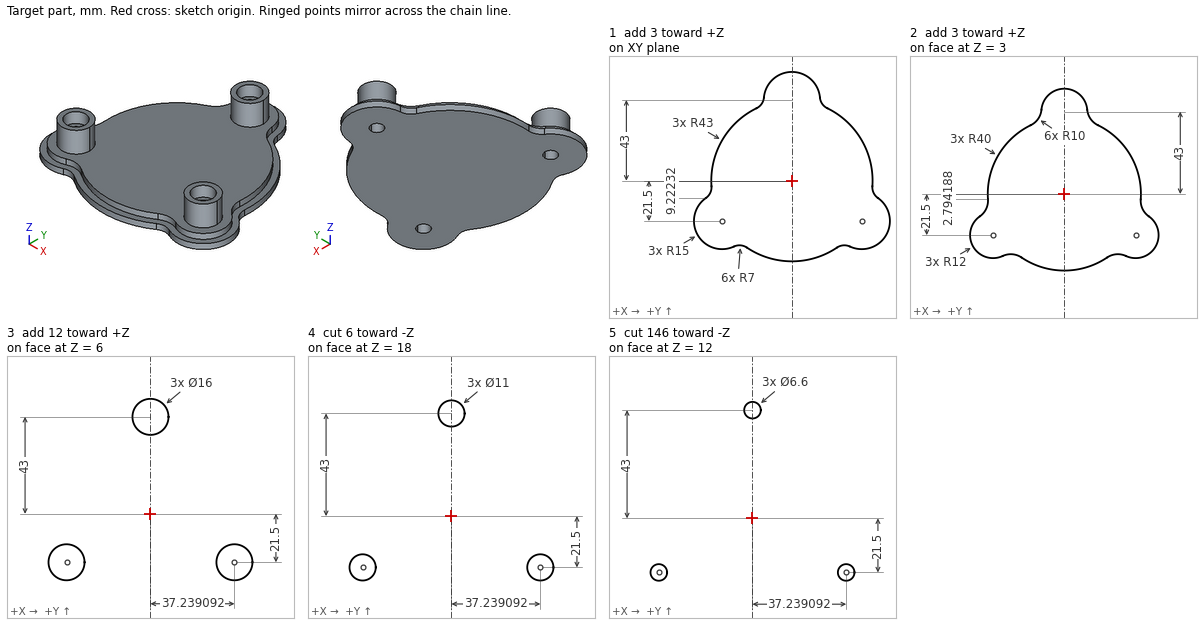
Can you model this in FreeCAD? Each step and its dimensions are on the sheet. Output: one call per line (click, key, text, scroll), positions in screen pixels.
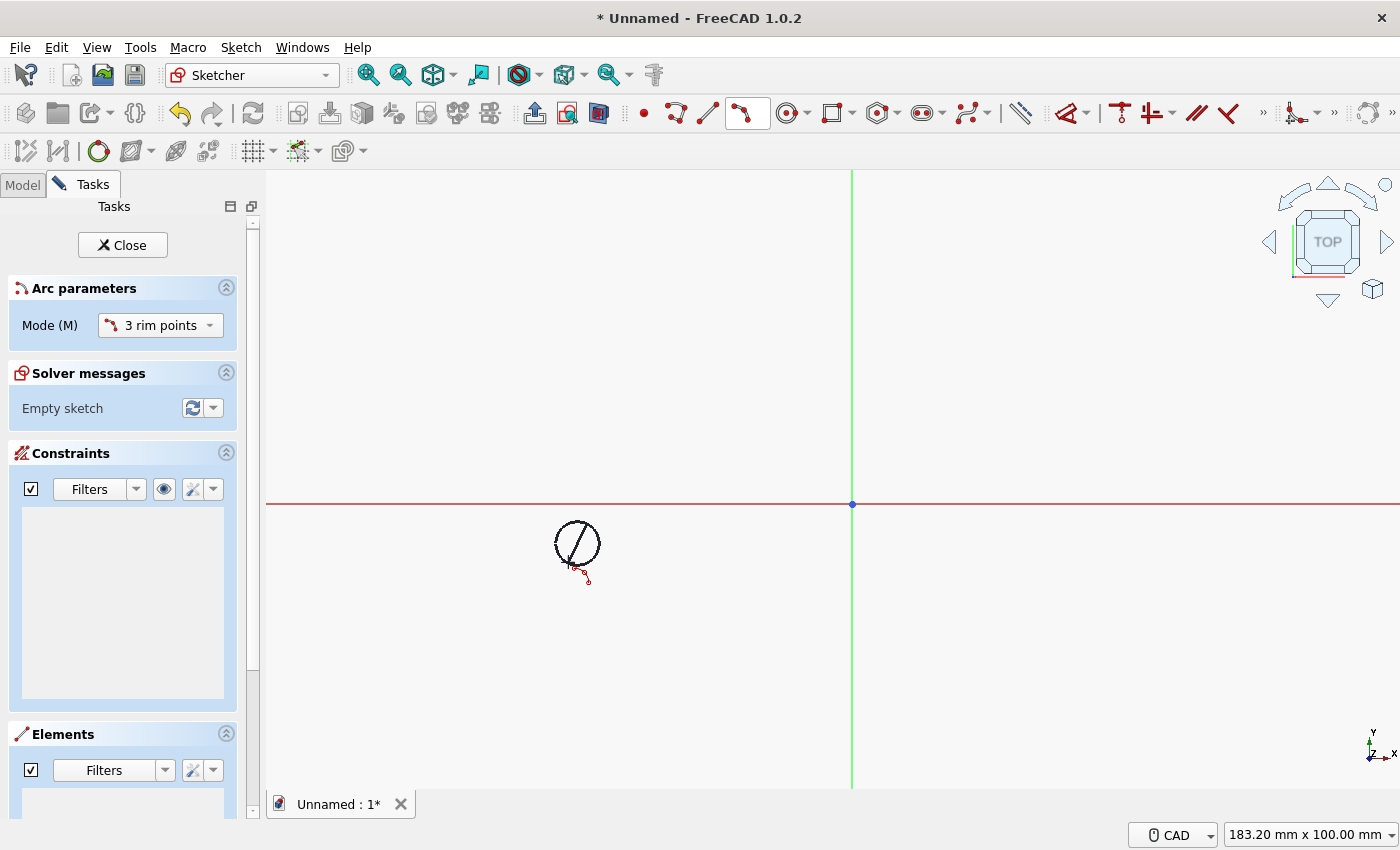
scroll(582, 545, up, 6)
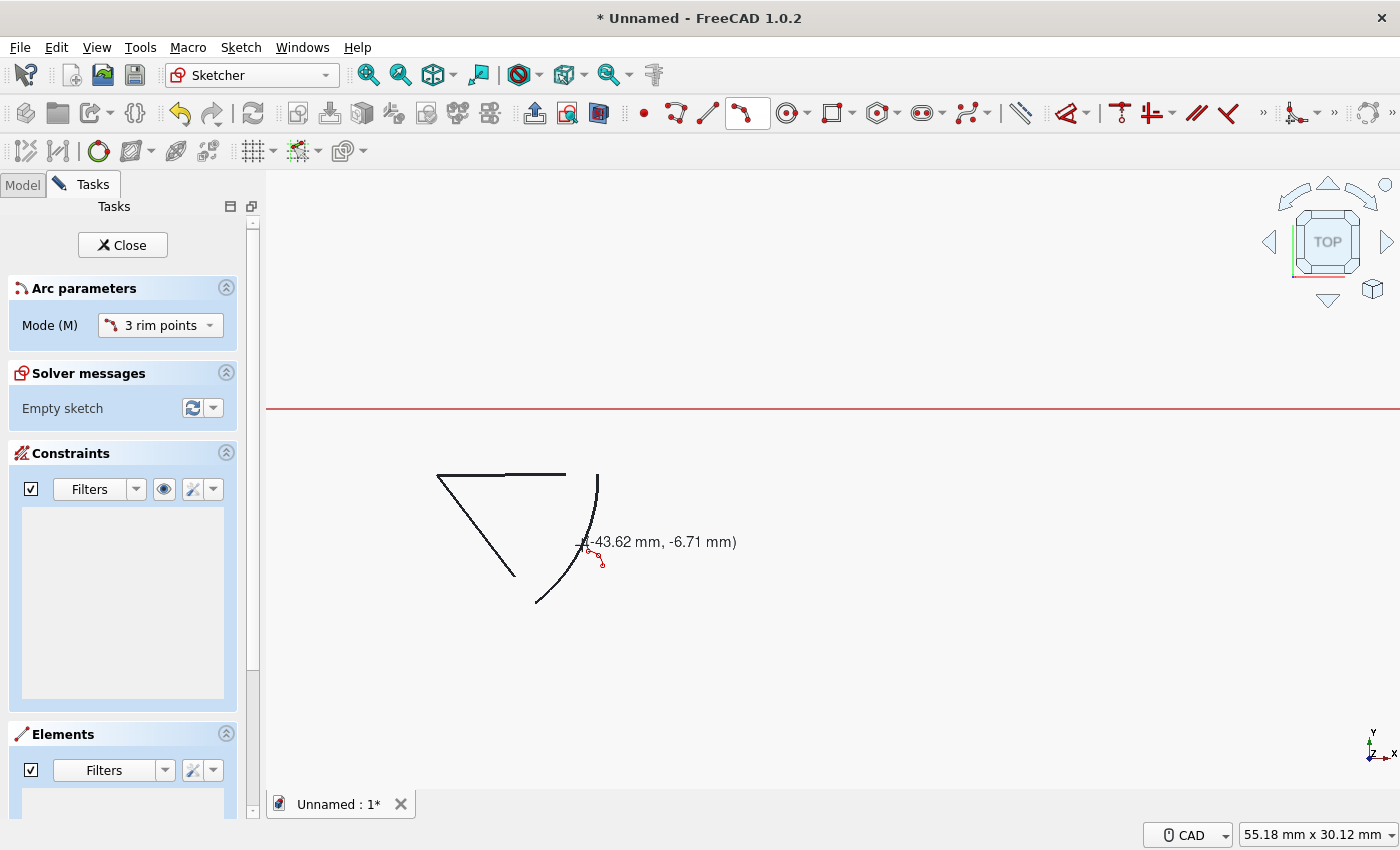
click(583, 543)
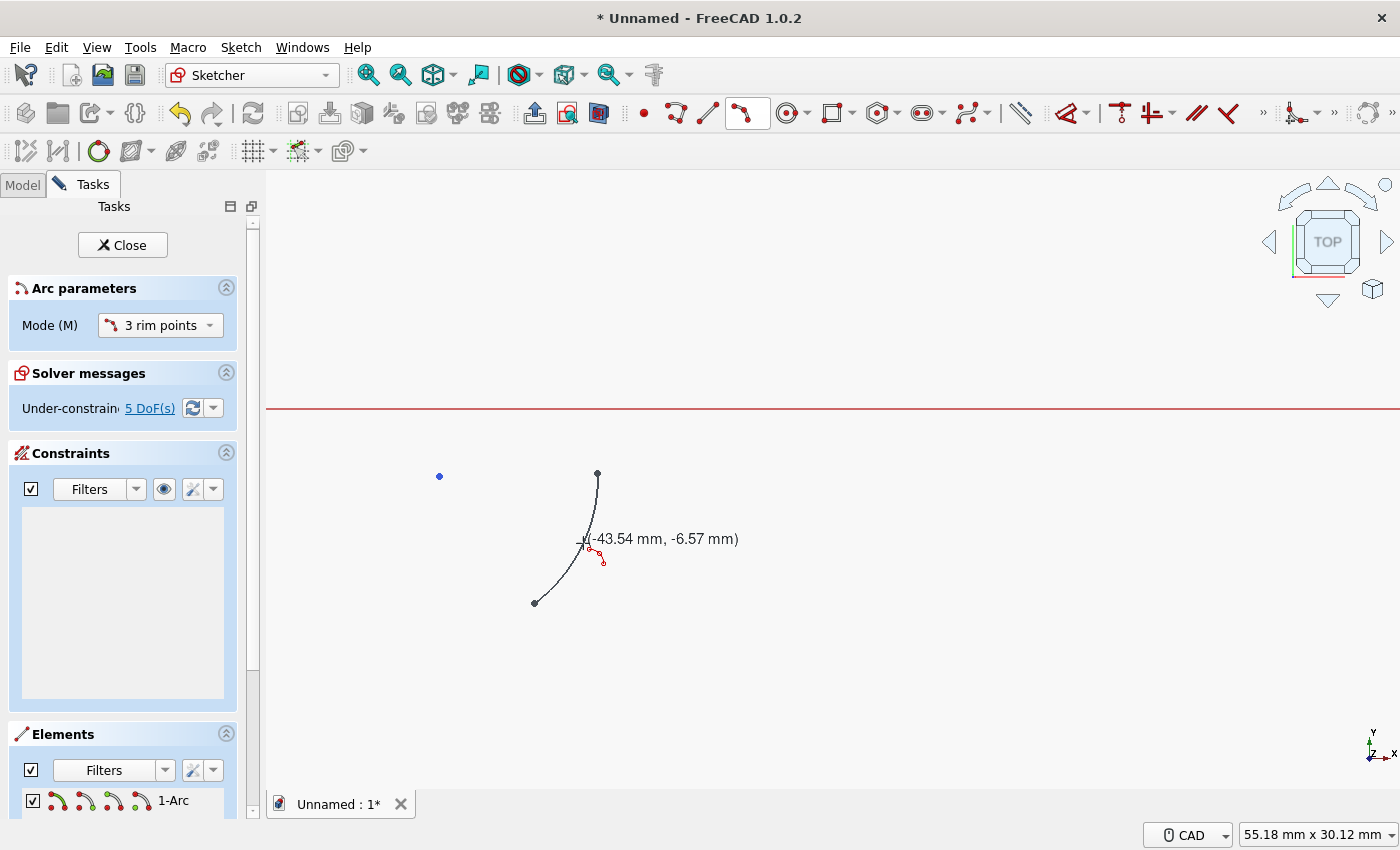
scroll(584, 536, down, 8)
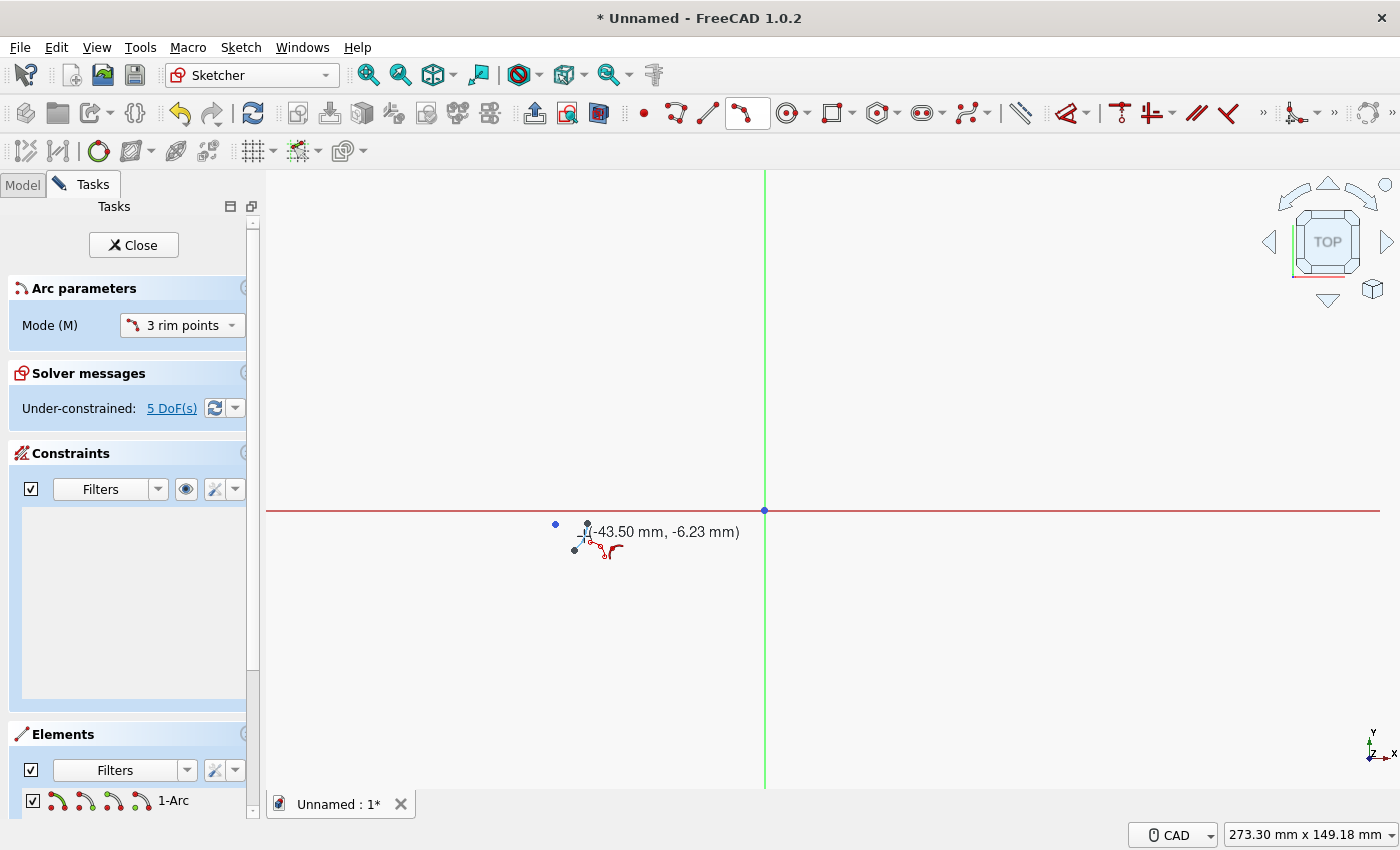
click(574, 550)
click(636, 656)
click(556, 631)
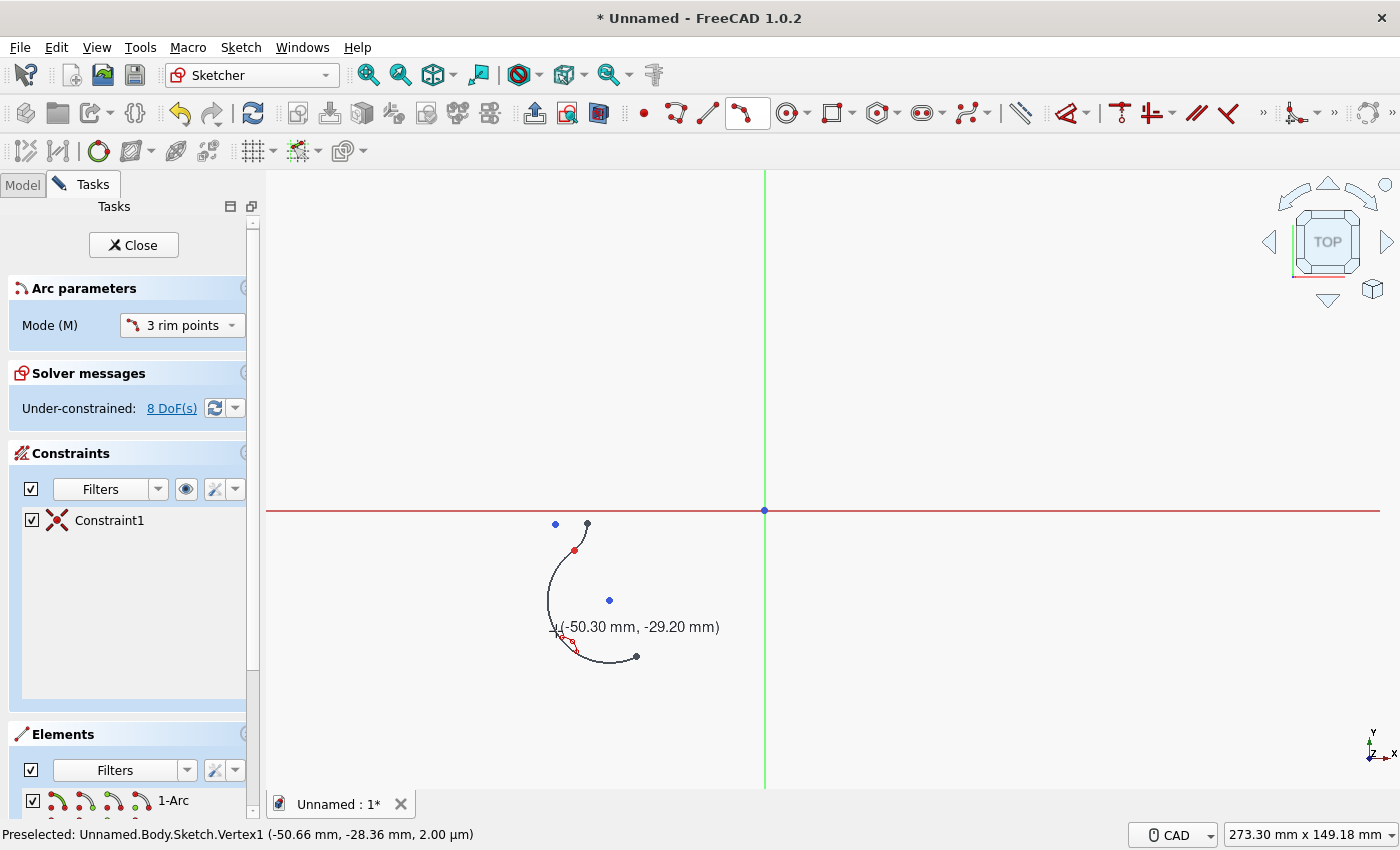
click(636, 657)
click(665, 659)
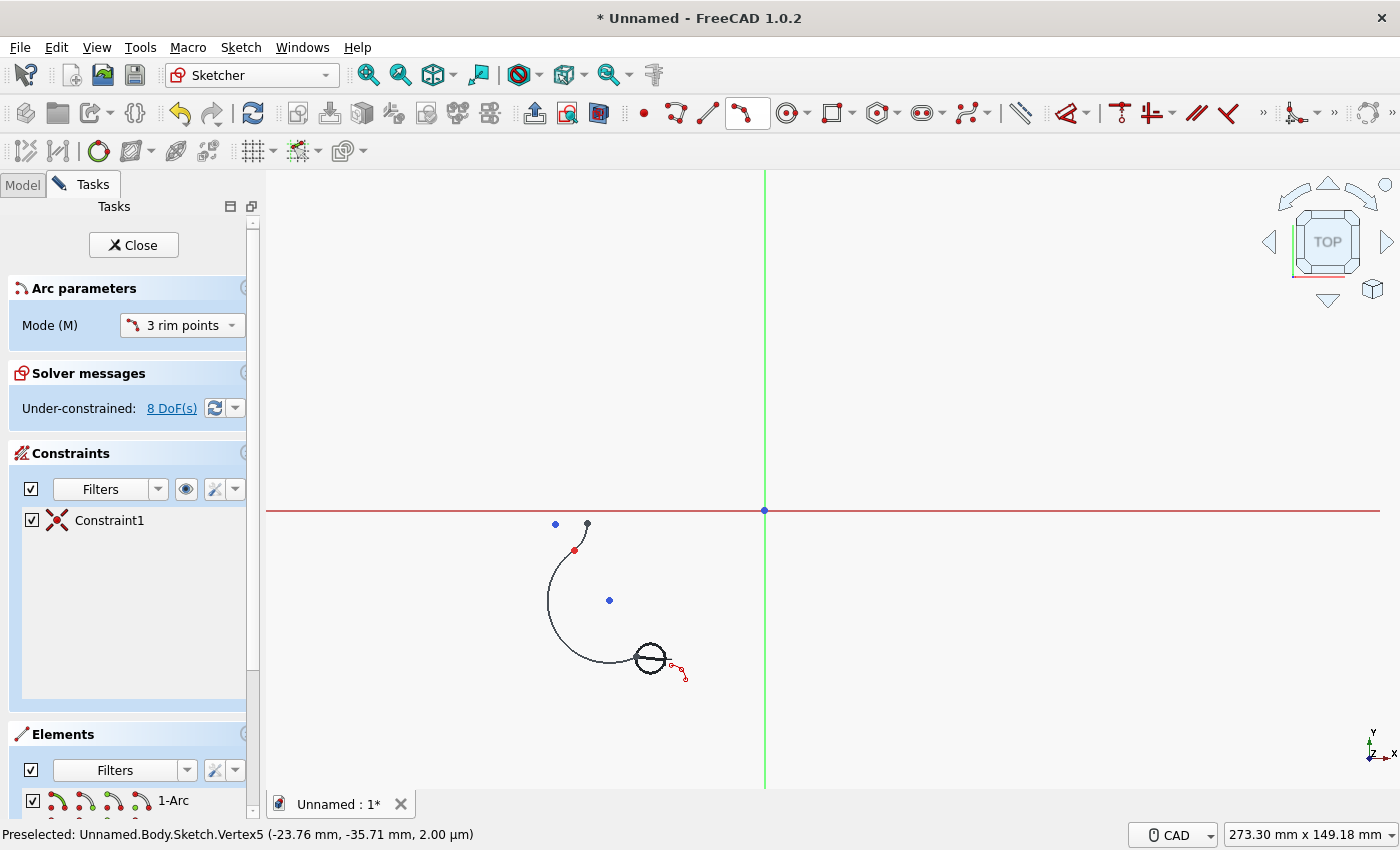
scroll(651, 654, up, 8)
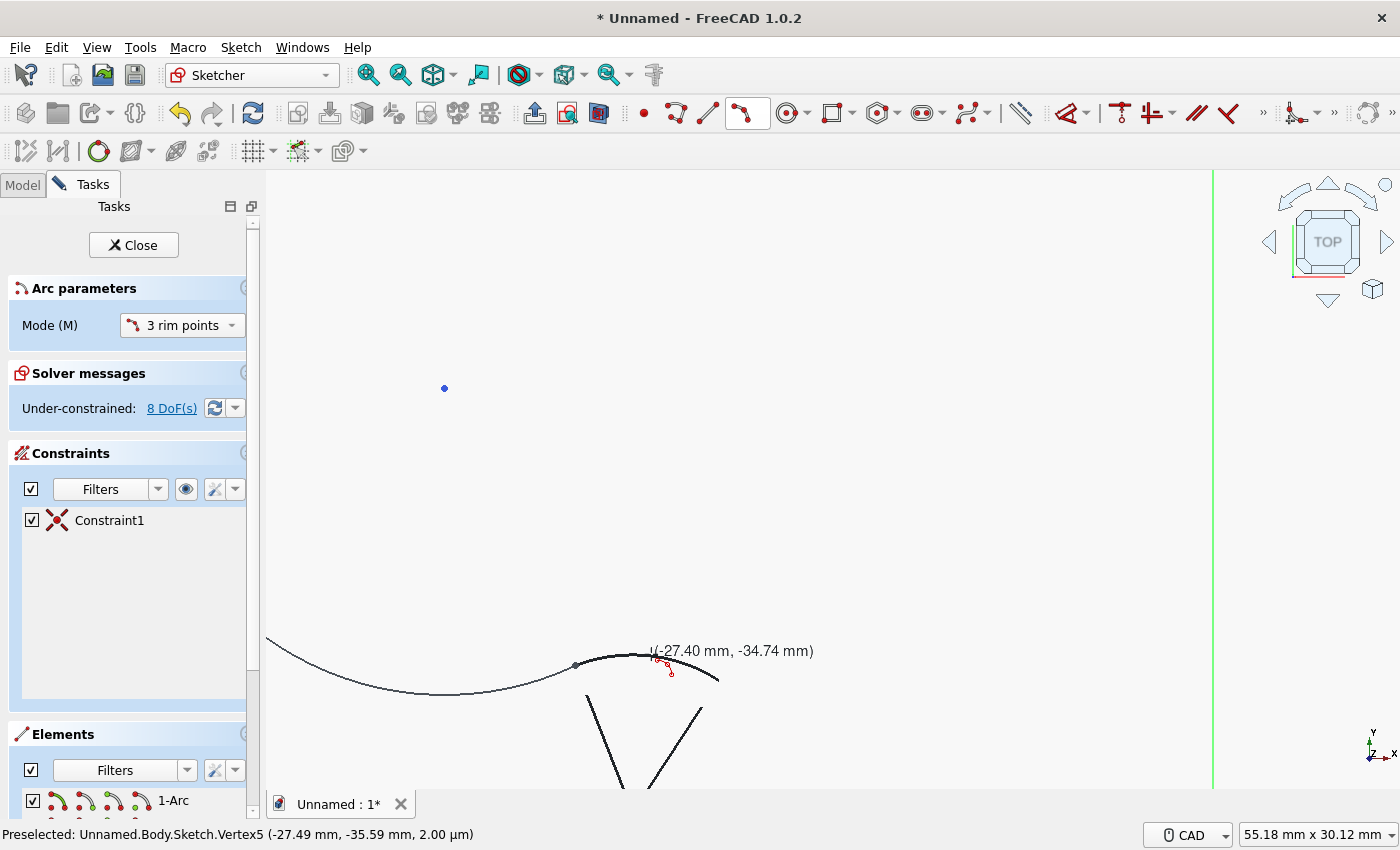
click(649, 650)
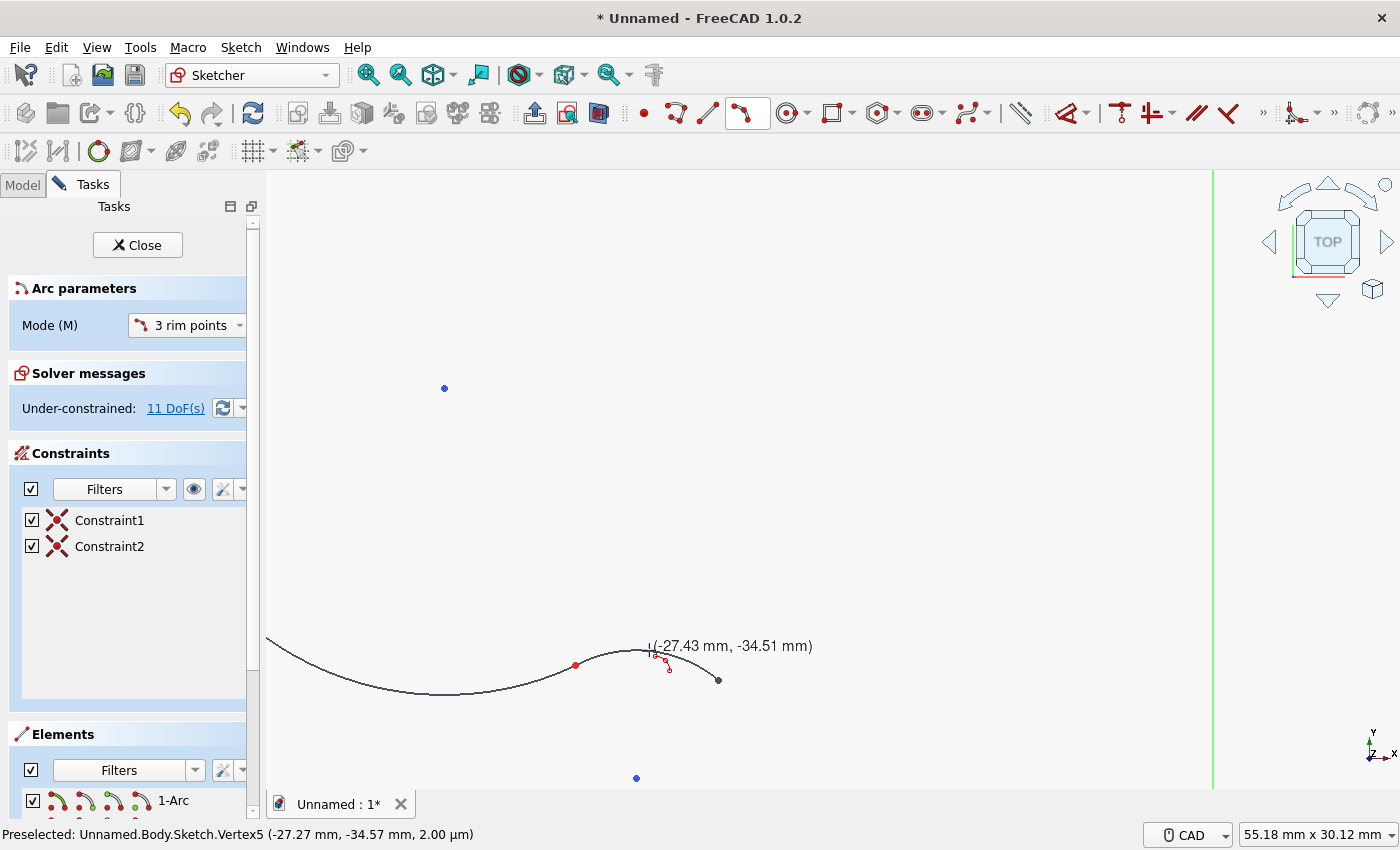
scroll(651, 655, down, 8)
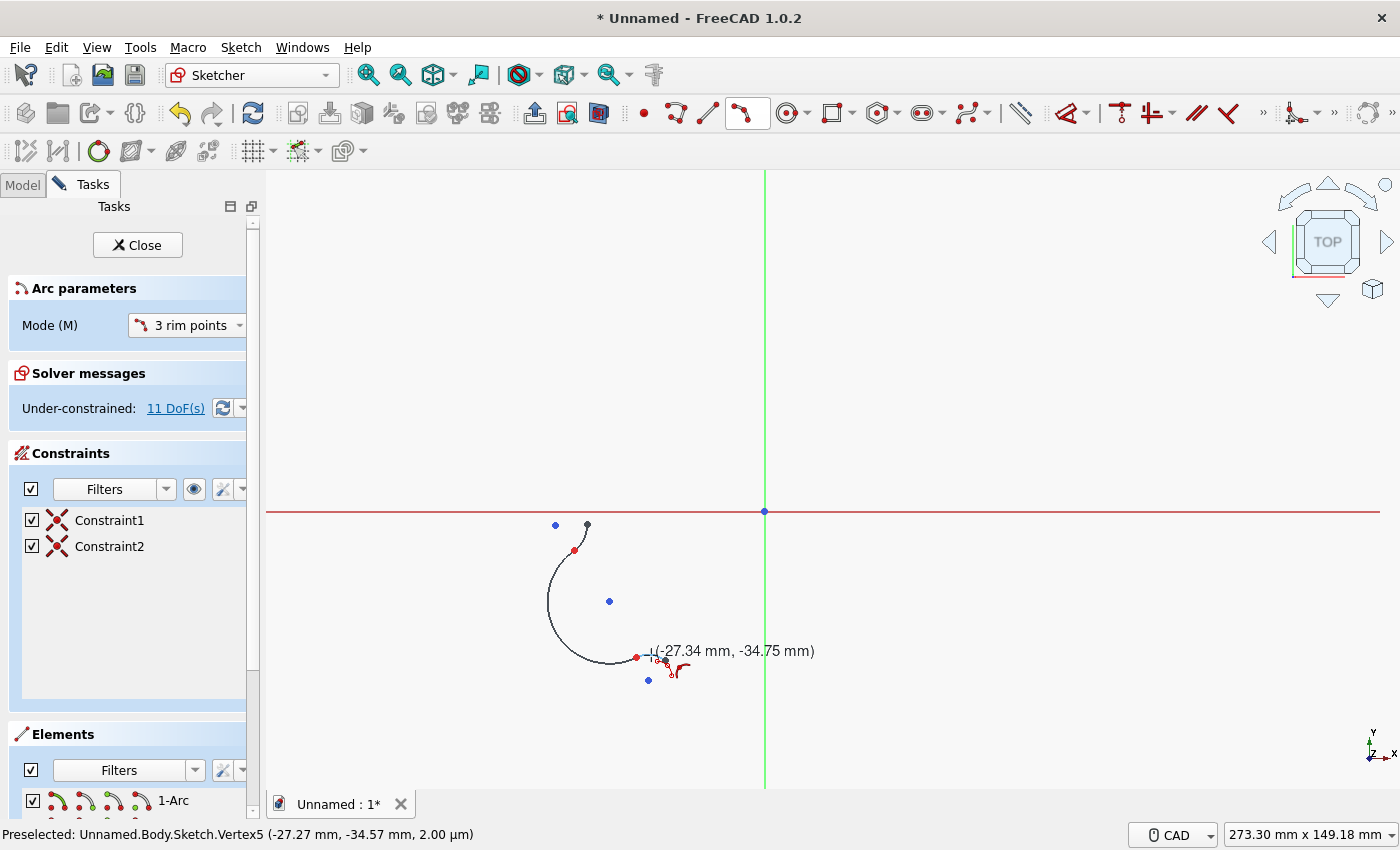
click(665, 661)
click(864, 660)
click(744, 689)